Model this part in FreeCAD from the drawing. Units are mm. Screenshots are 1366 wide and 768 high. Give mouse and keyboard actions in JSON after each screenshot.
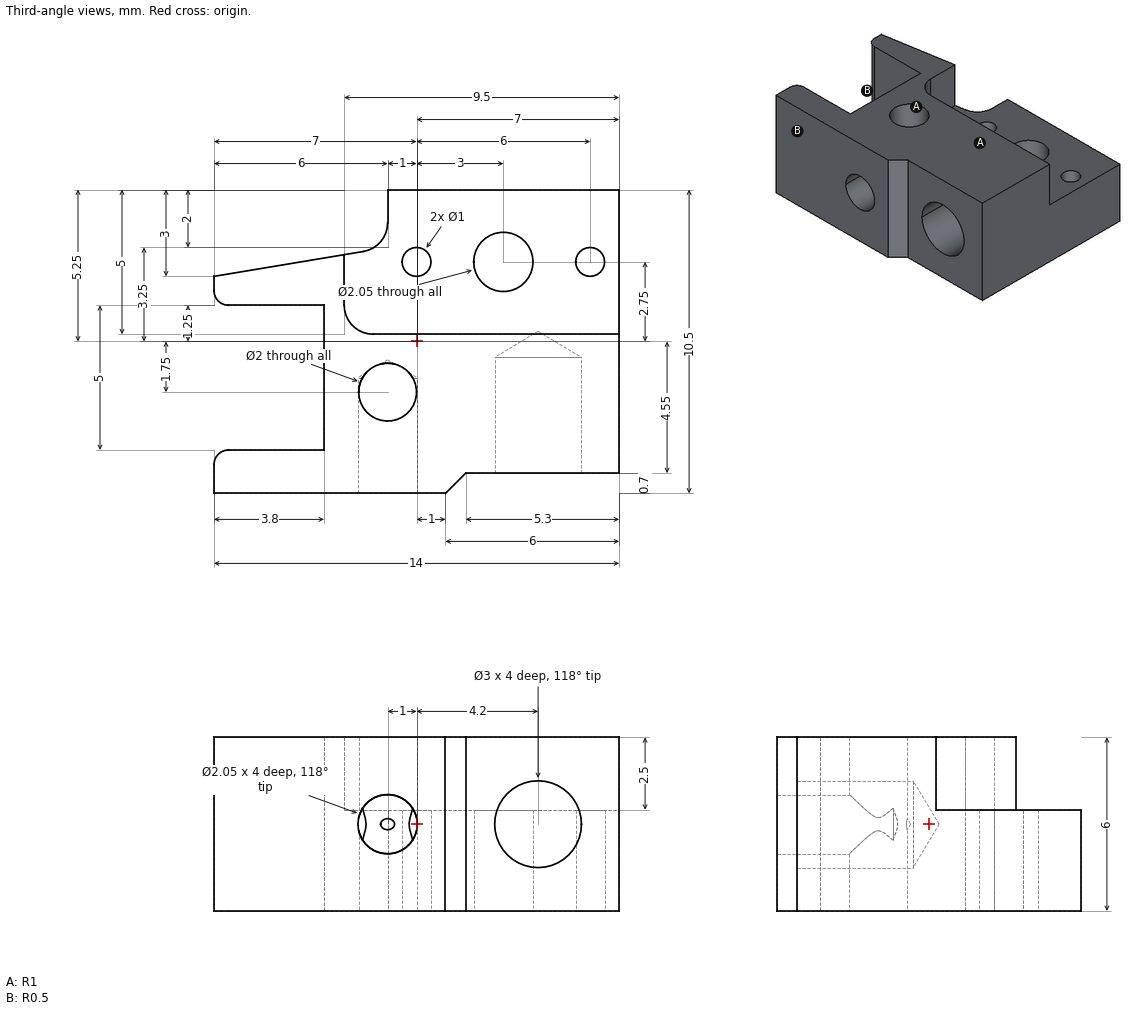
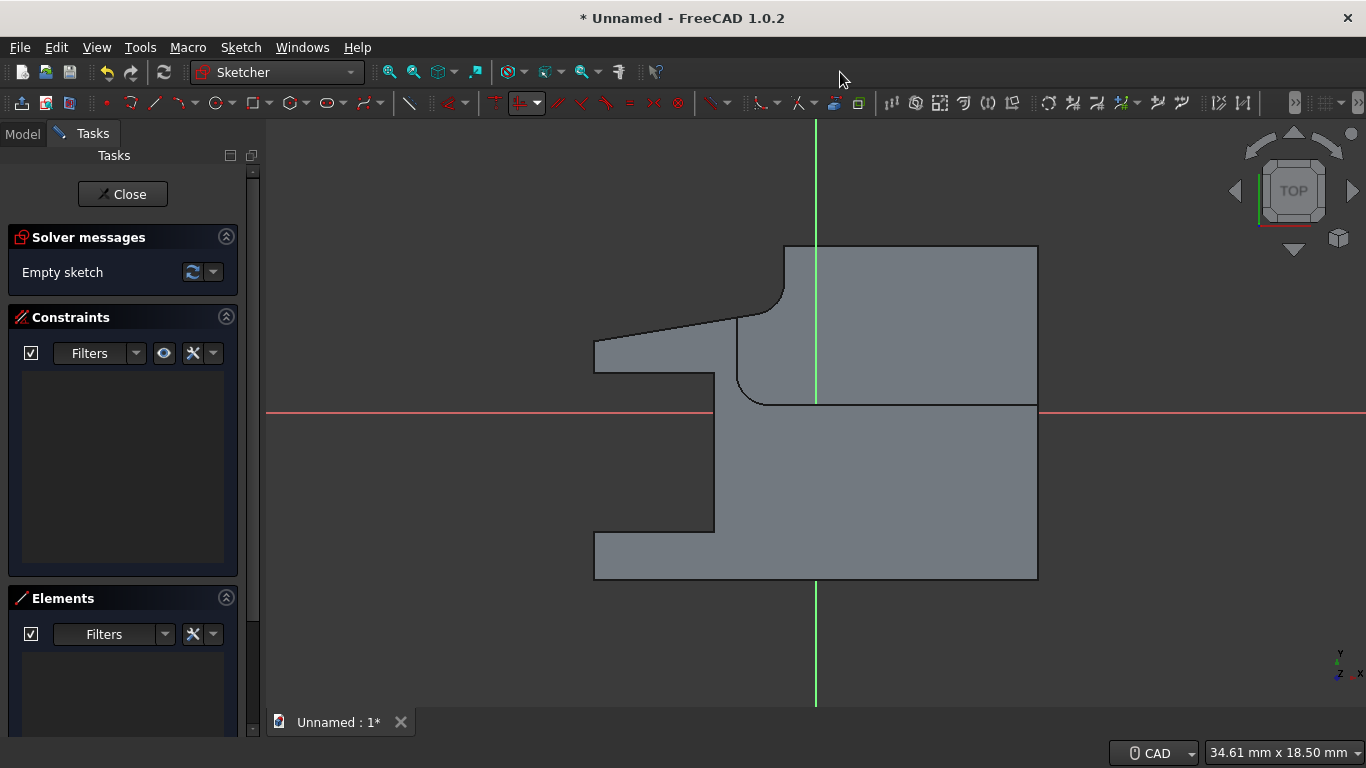
{"action": "scroll", "coordinate": [937, 327], "scroll_direction": "up", "scroll_amount": 6}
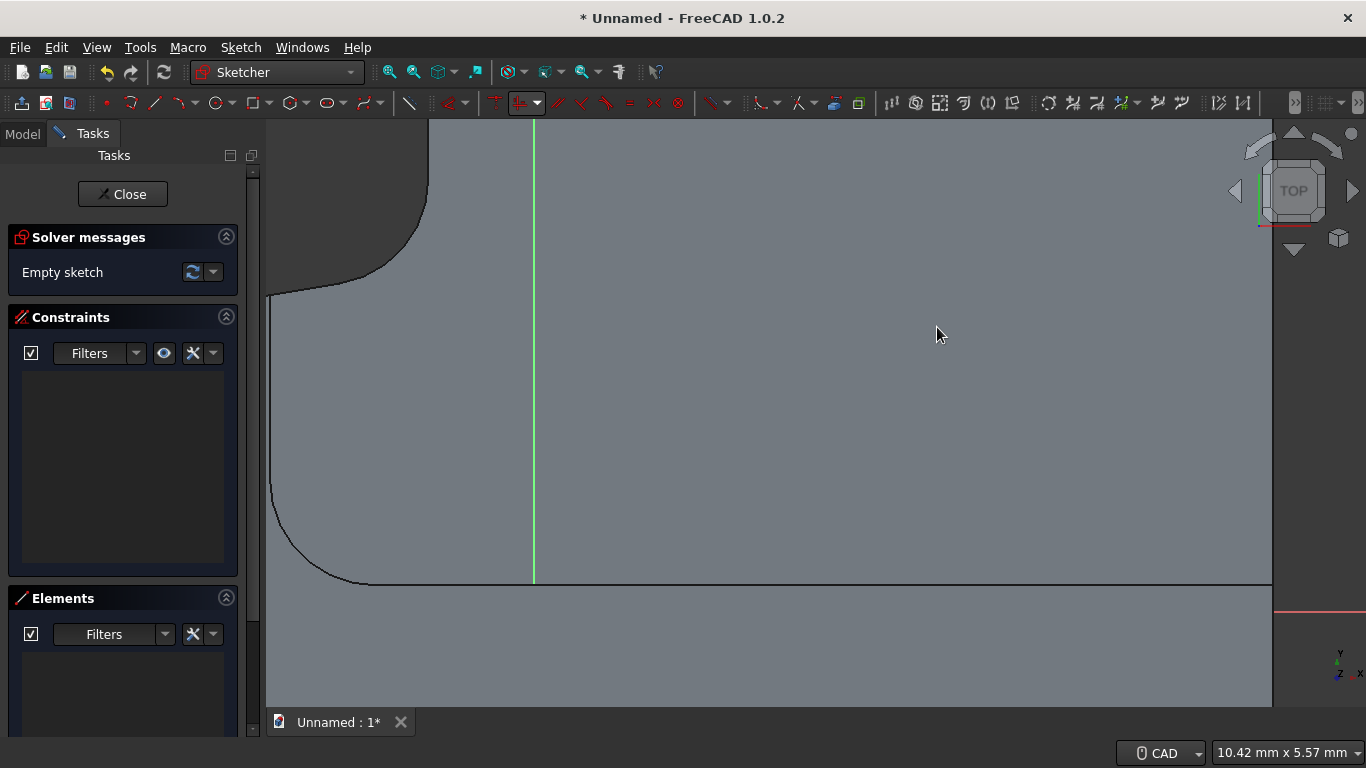
{"action": "left_click", "coordinate": [216, 104]}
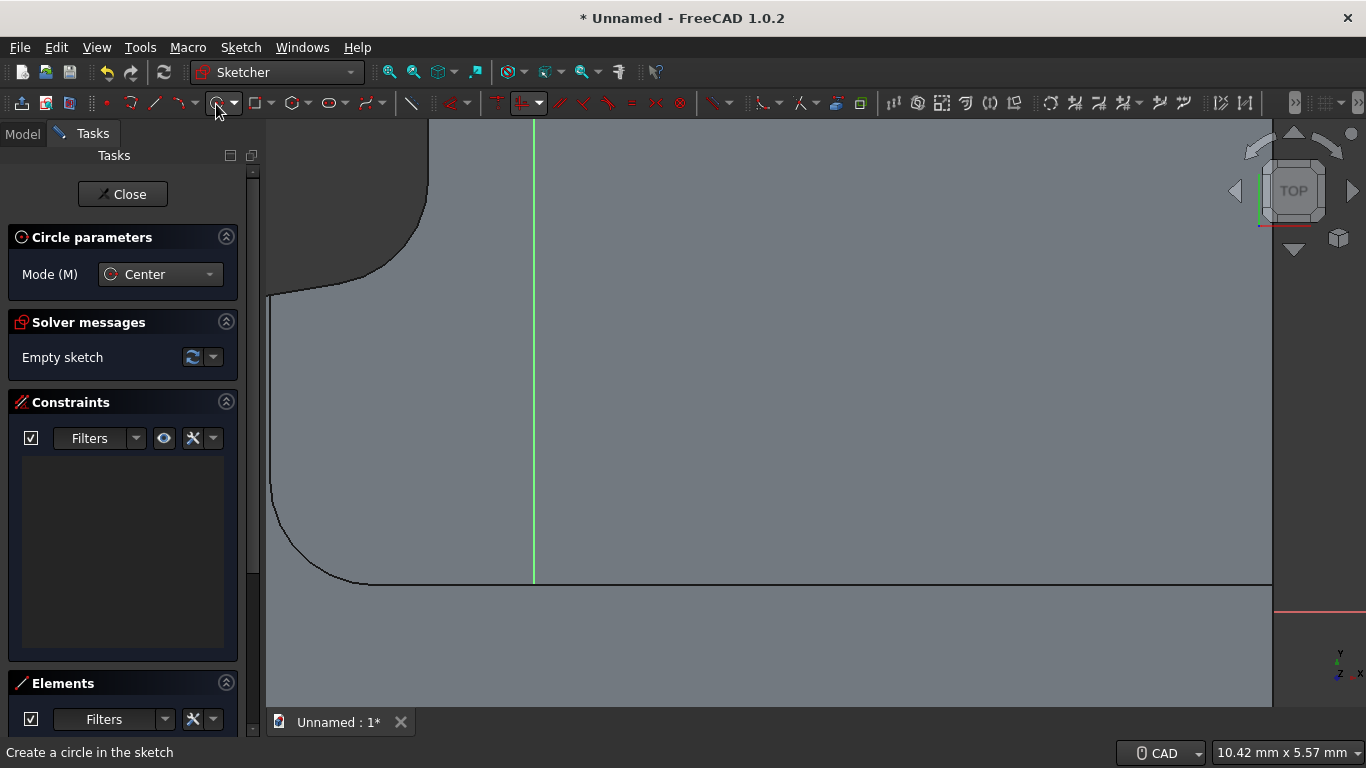
{"action": "left_click", "coordinate": [850, 322]}
{"action": "left_click", "coordinate": [927, 245]}
{"action": "key", "text": "Escape"}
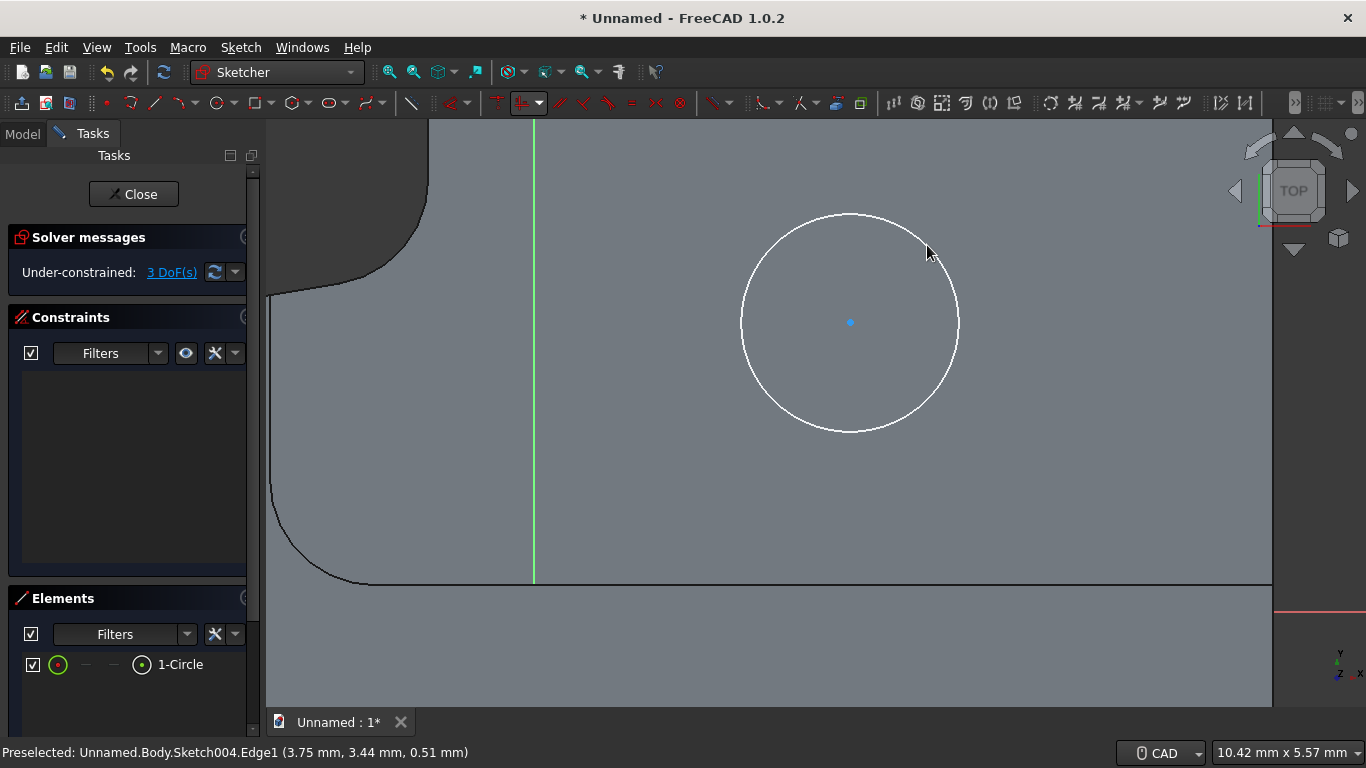
{"action": "left_click", "coordinate": [450, 104]}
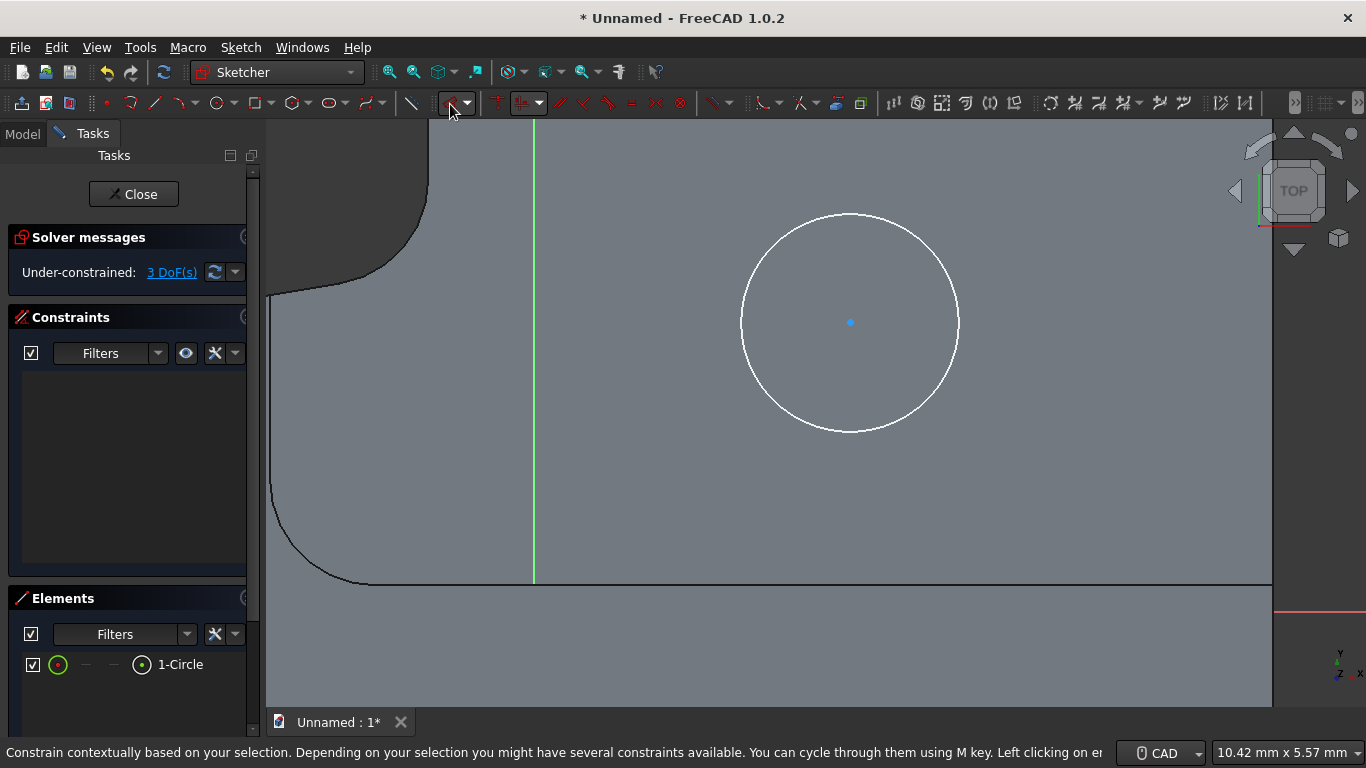
{"action": "left_click", "coordinate": [927, 246]}
{"action": "left_click", "coordinate": [950, 223]}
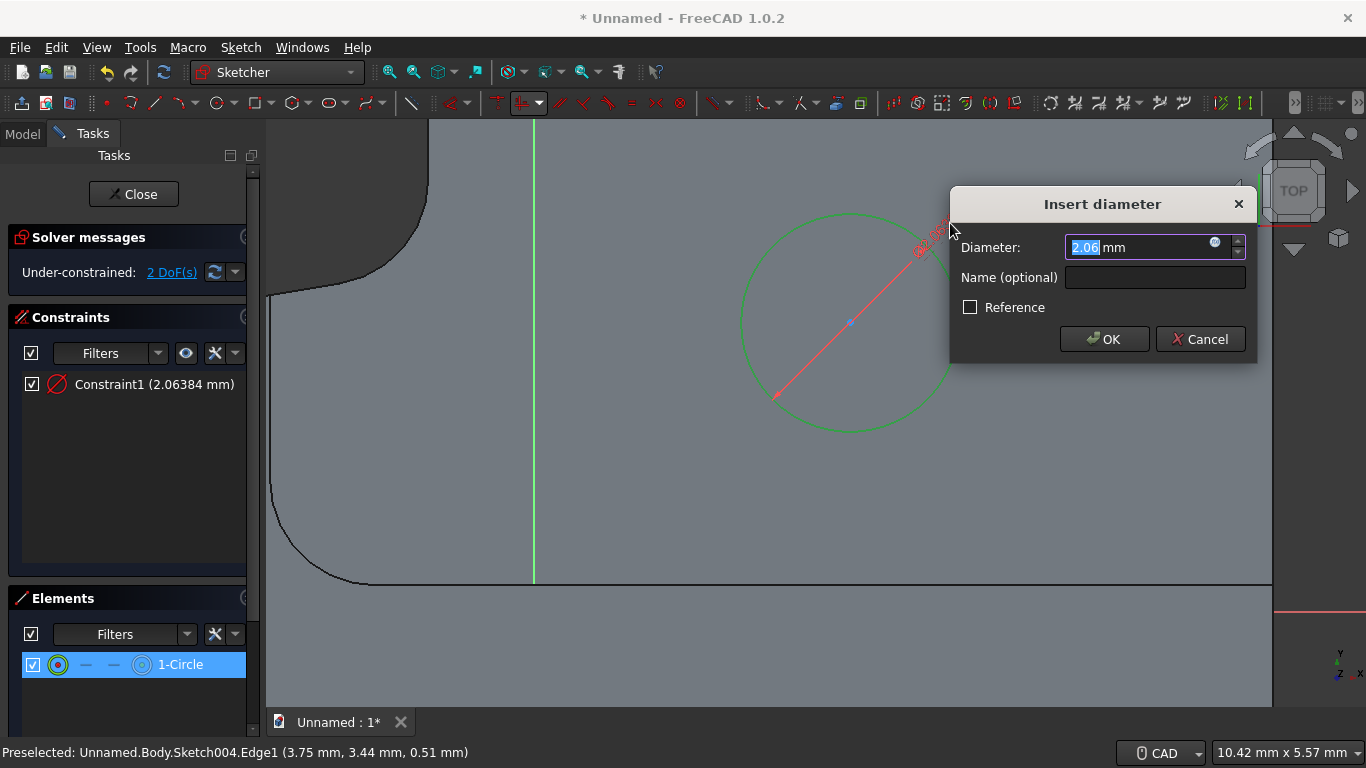
{"action": "type", "text": "2.05"}
{"action": "key", "text": "Return"}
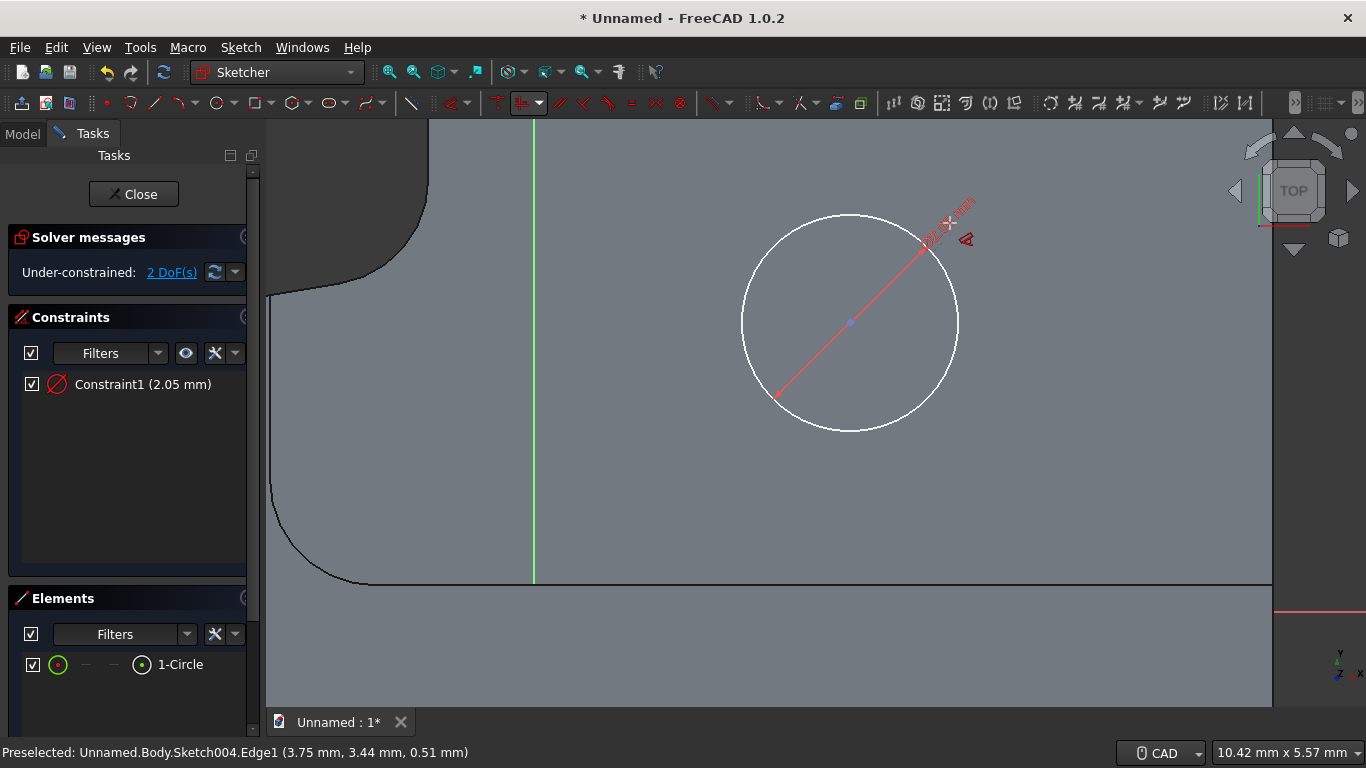
{"action": "left_click", "coordinate": [850, 323]}
{"action": "left_click", "coordinate": [692, 646]}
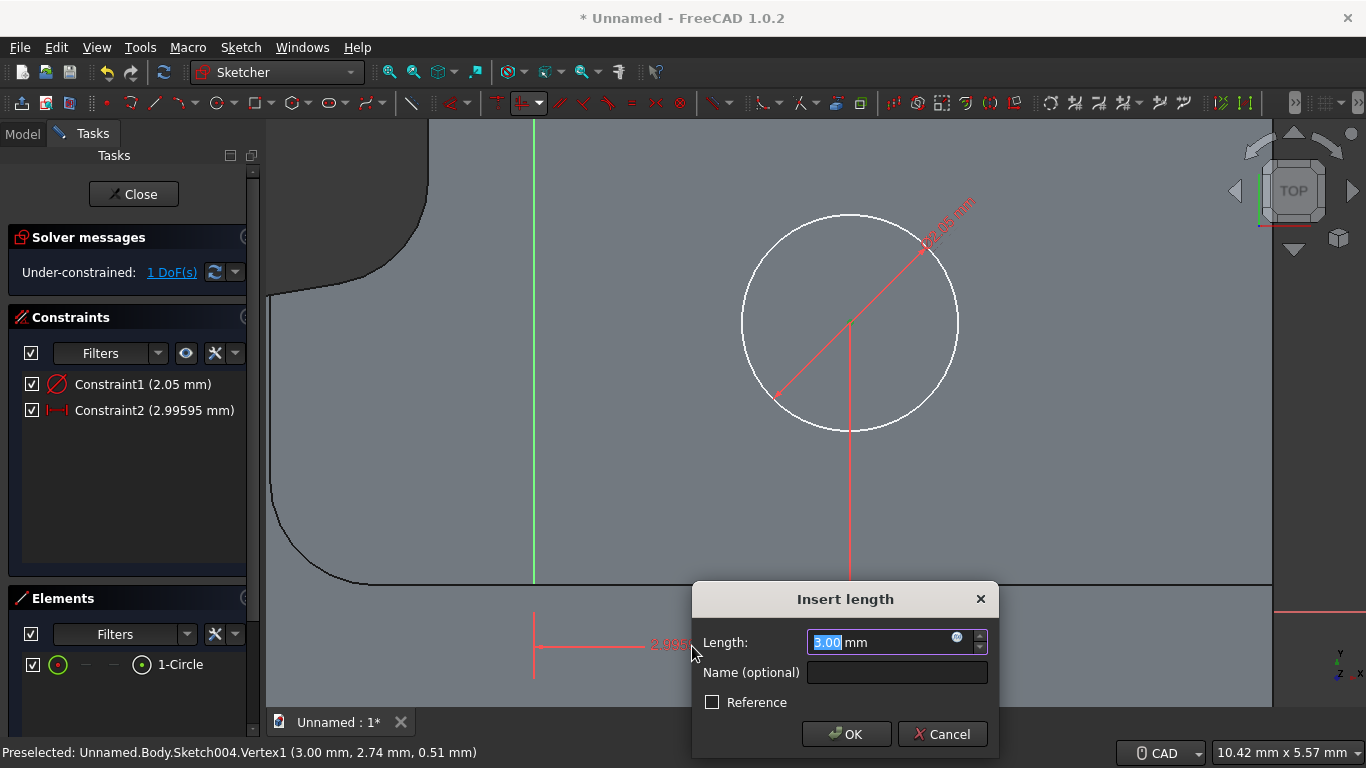
{"action": "type", "text": "3"}
{"action": "key", "text": "Return"}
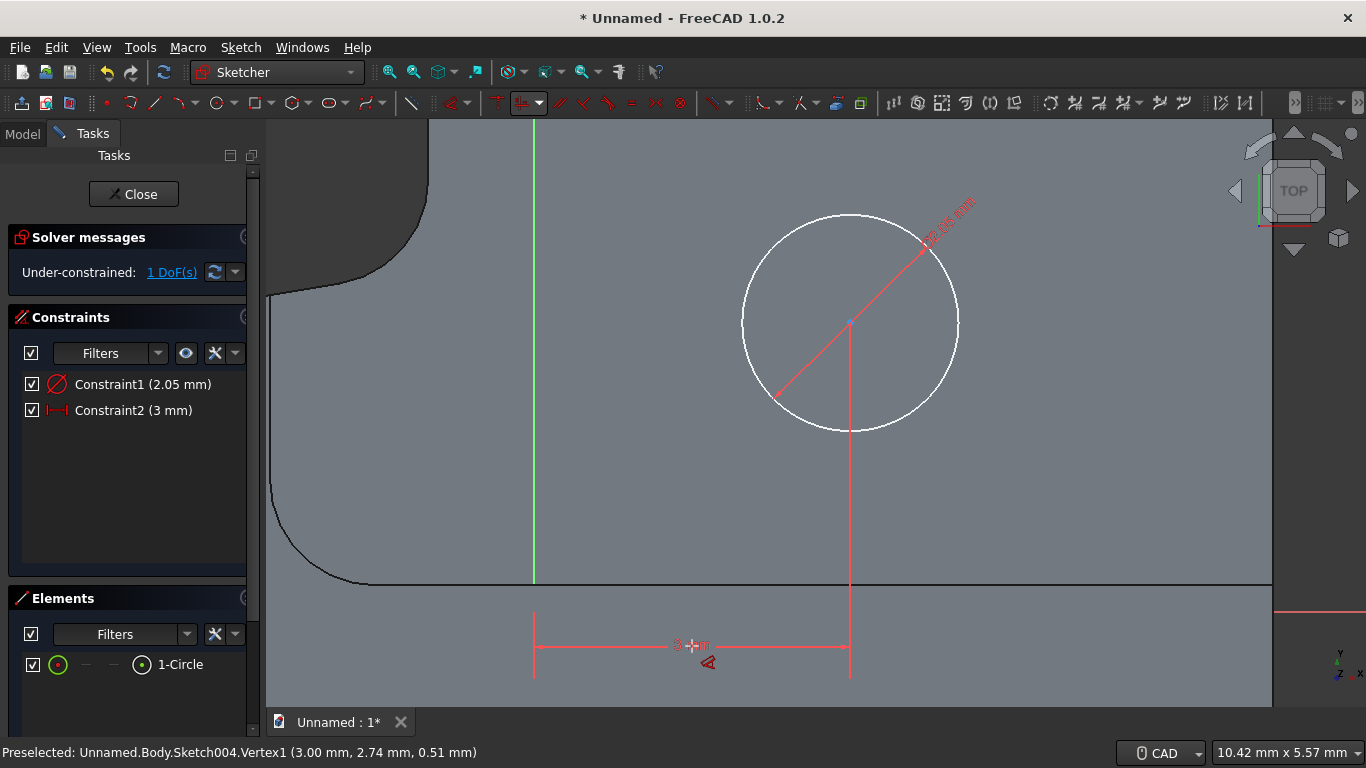
{"action": "left_click", "coordinate": [850, 323]}
{"action": "left_click", "coordinate": [500, 467]}